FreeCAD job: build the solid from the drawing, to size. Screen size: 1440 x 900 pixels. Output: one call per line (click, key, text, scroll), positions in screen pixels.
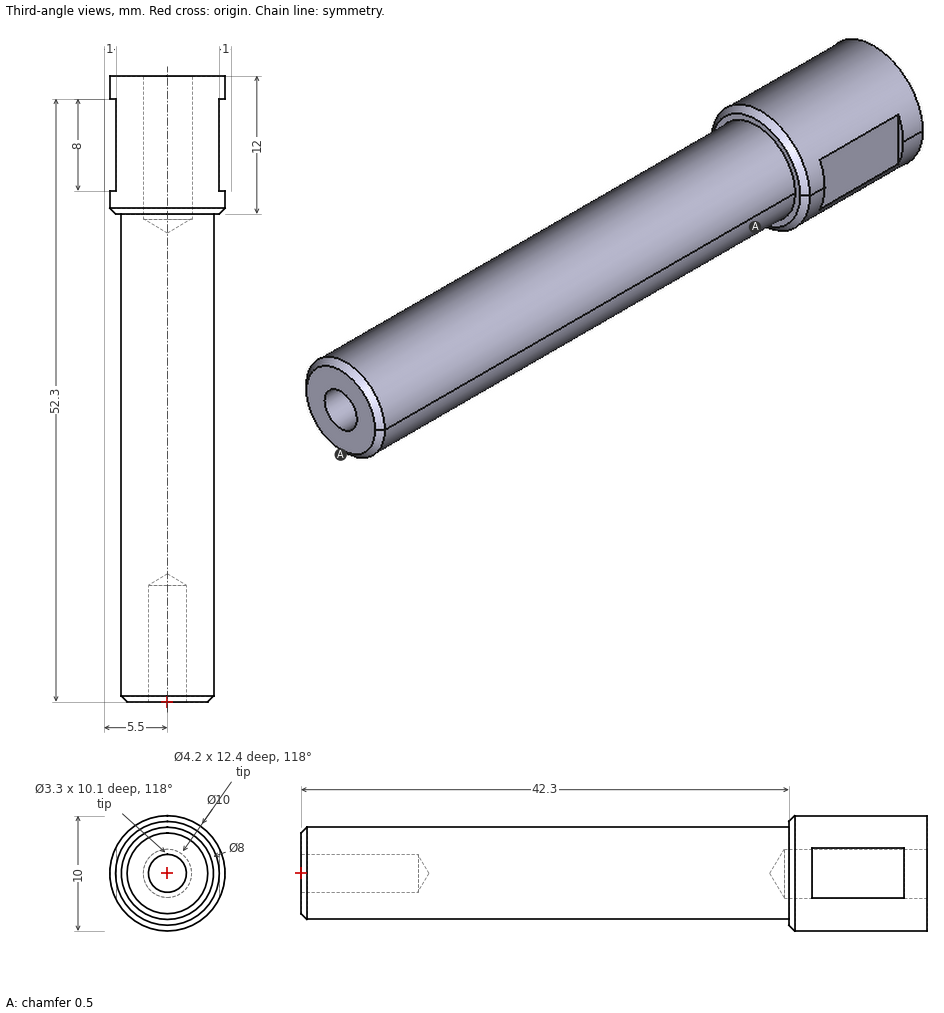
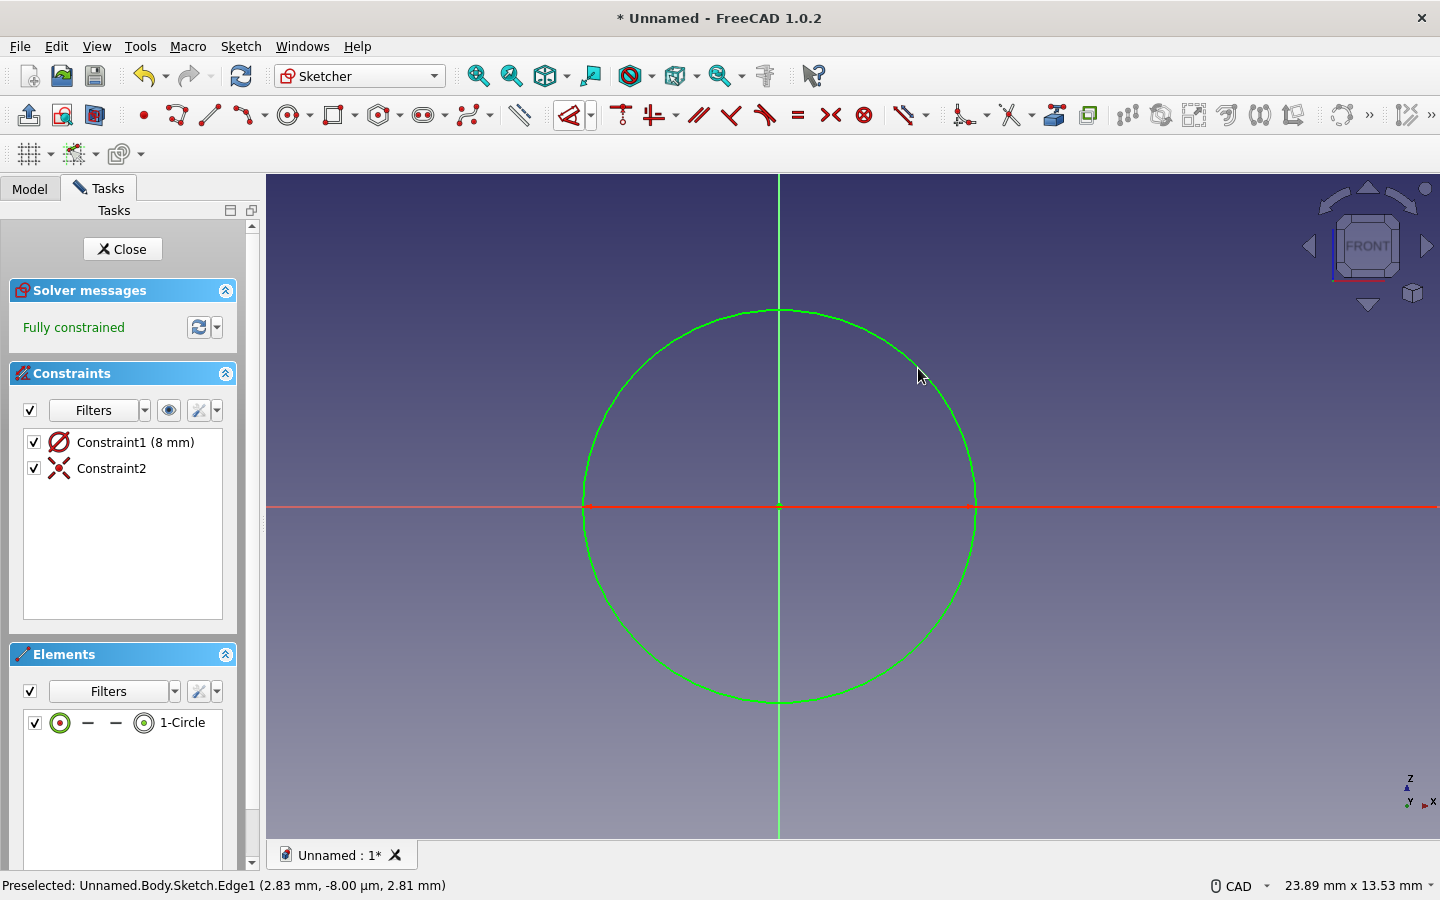
click(123, 249)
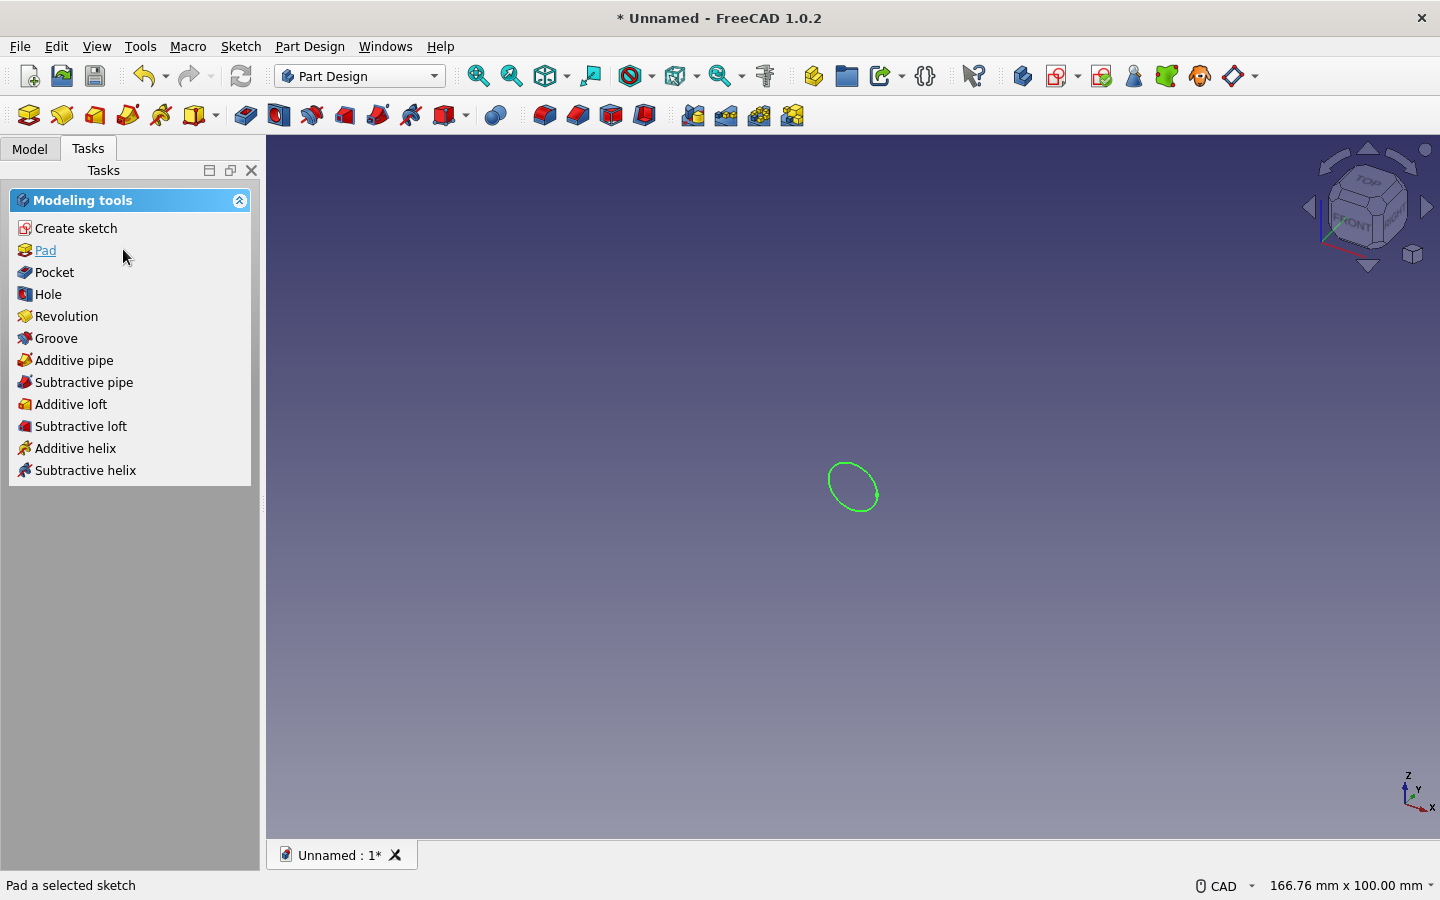
click(29, 116)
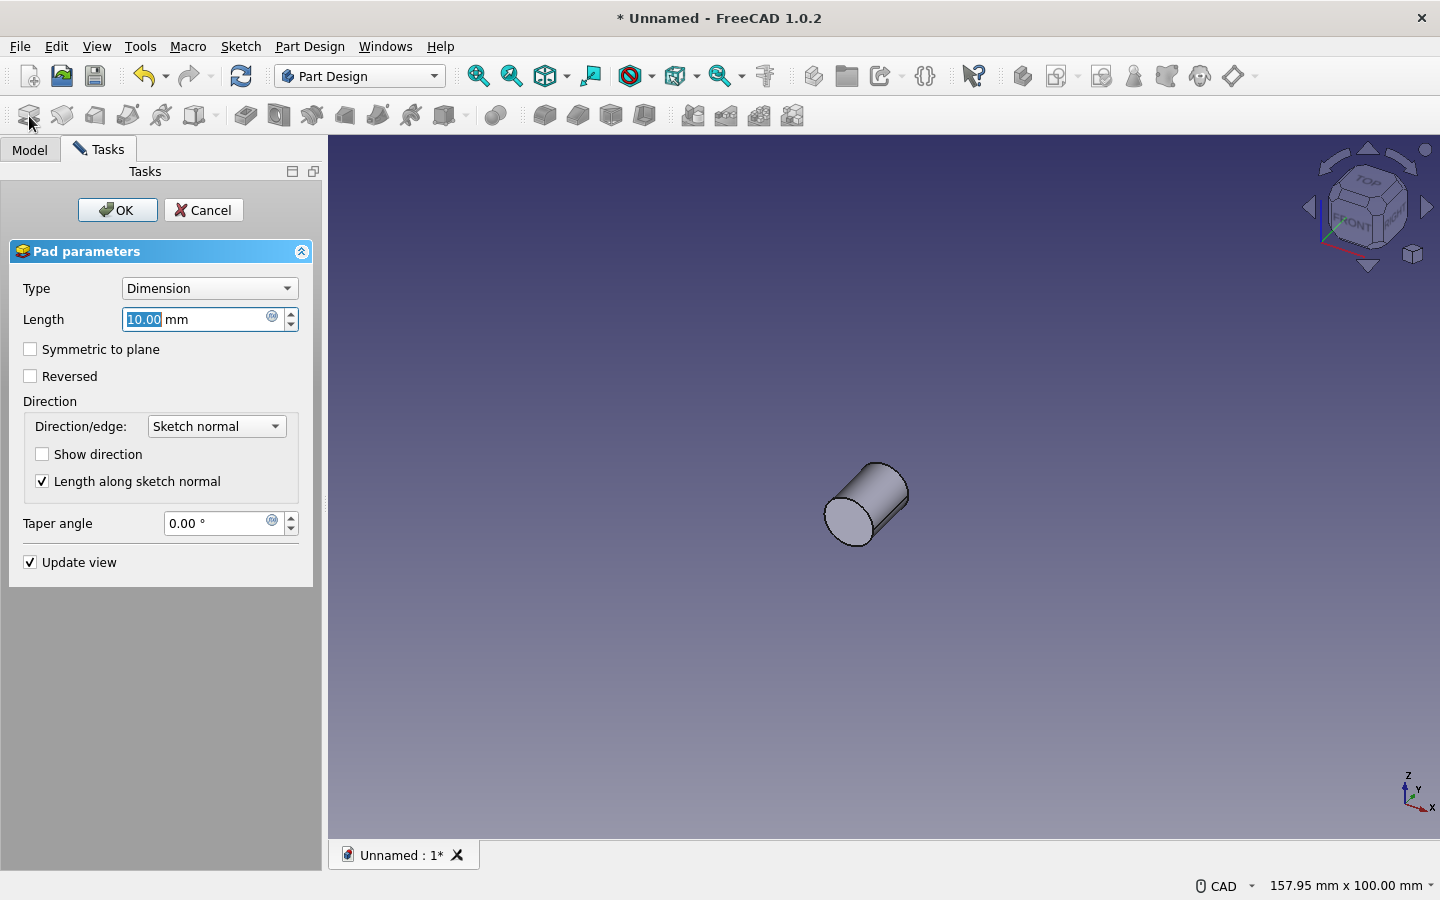
text(42.3)
key(Tab)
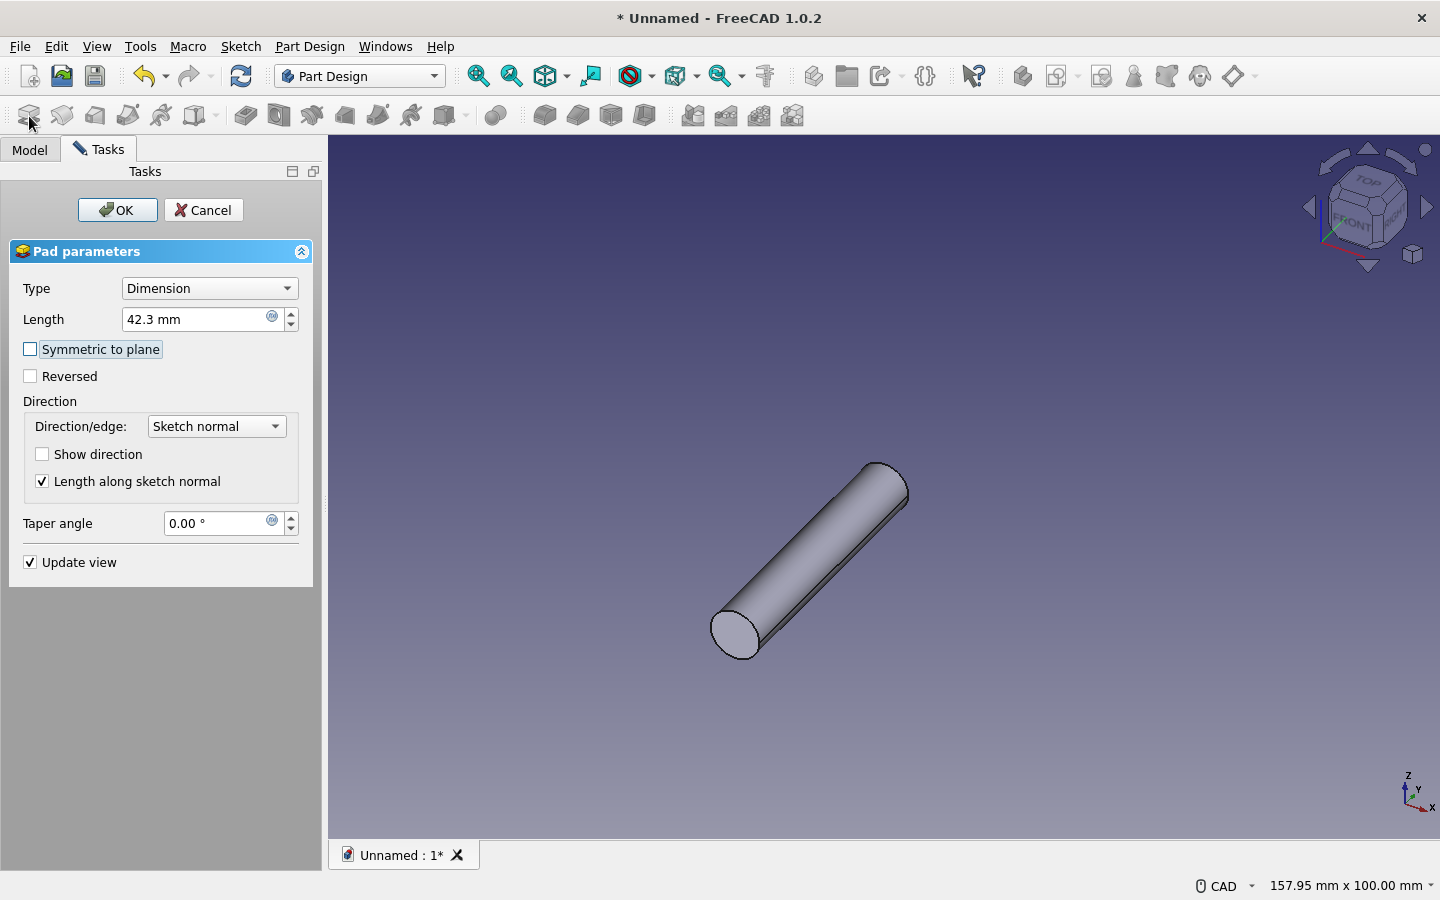
click(31, 376)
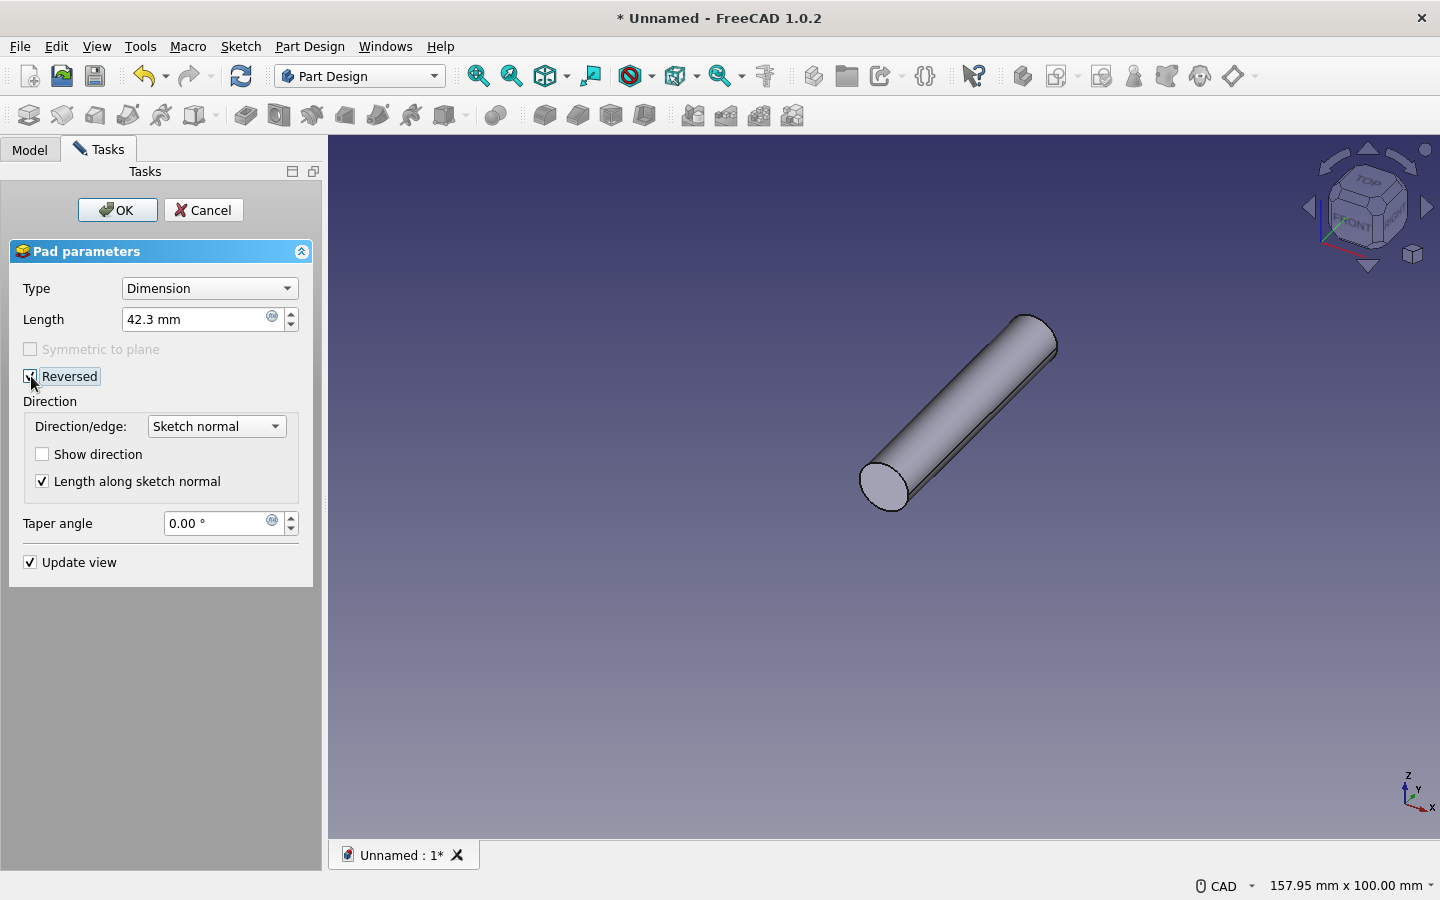
click(118, 210)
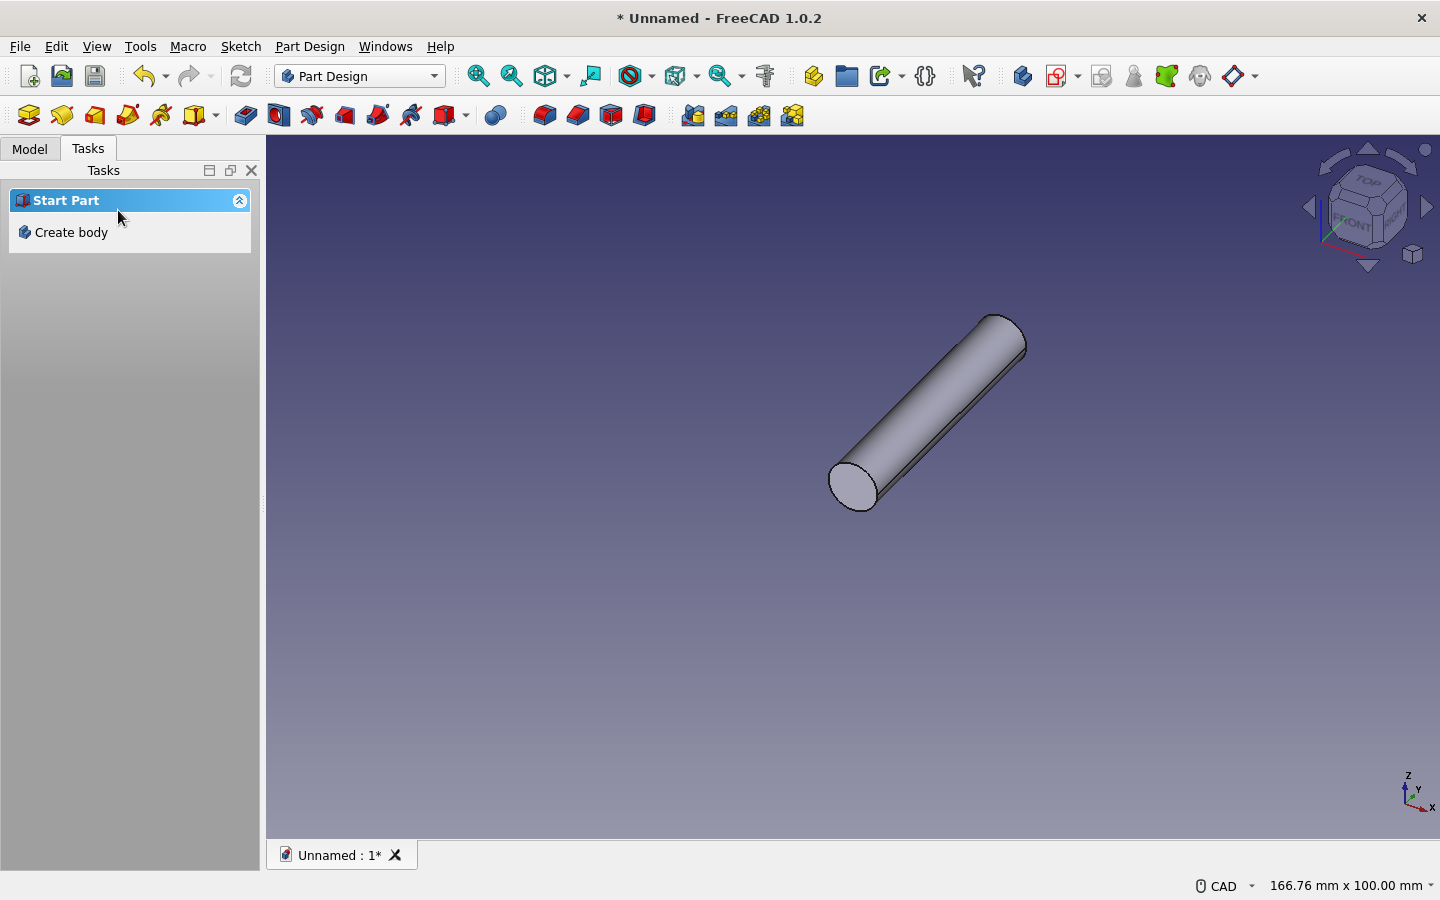
key(v)
key(f)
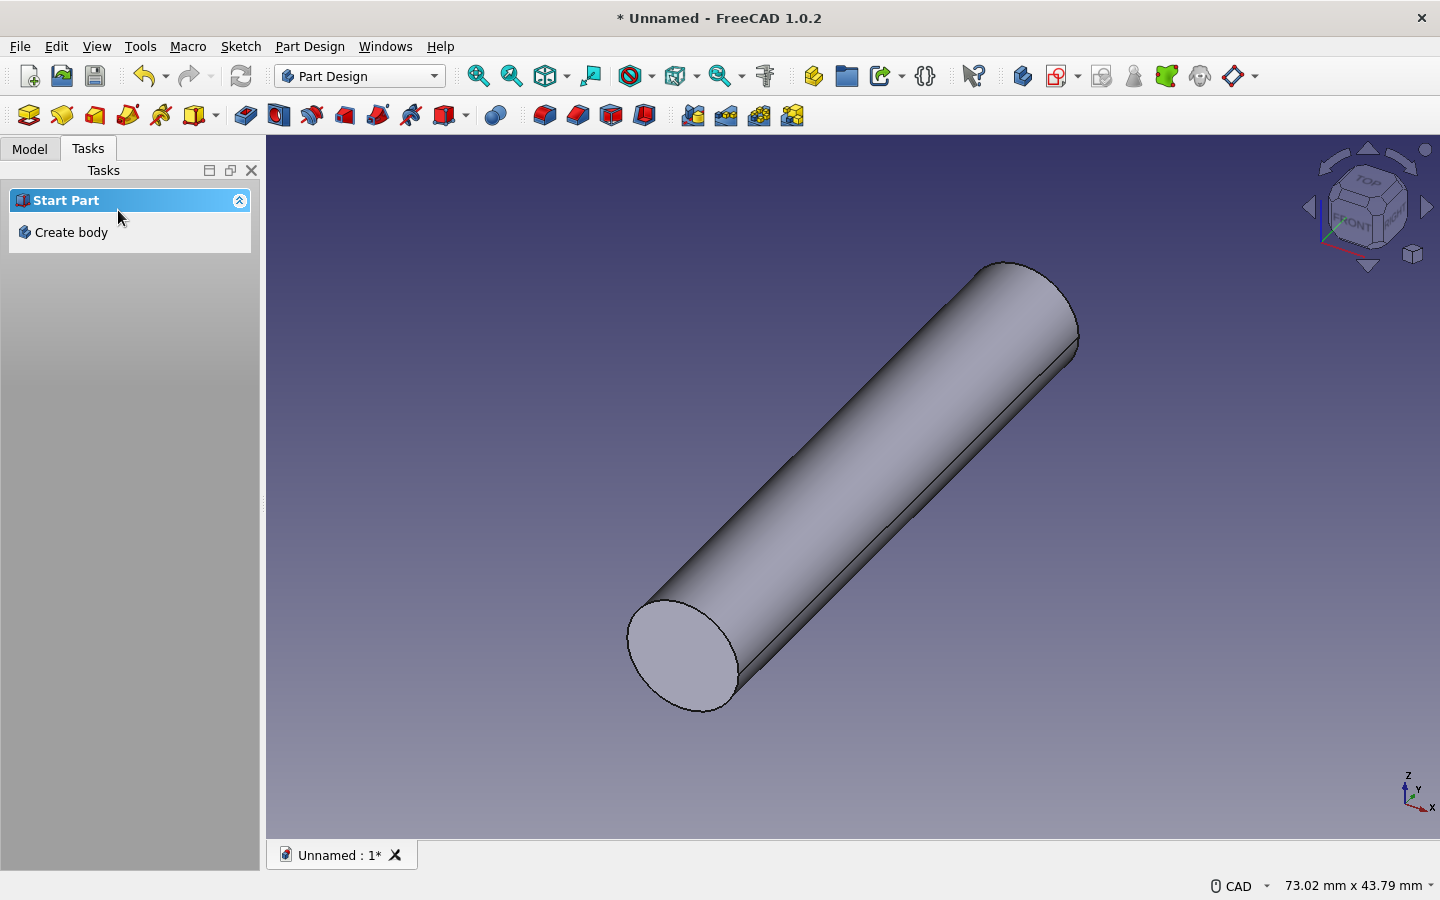
key(4)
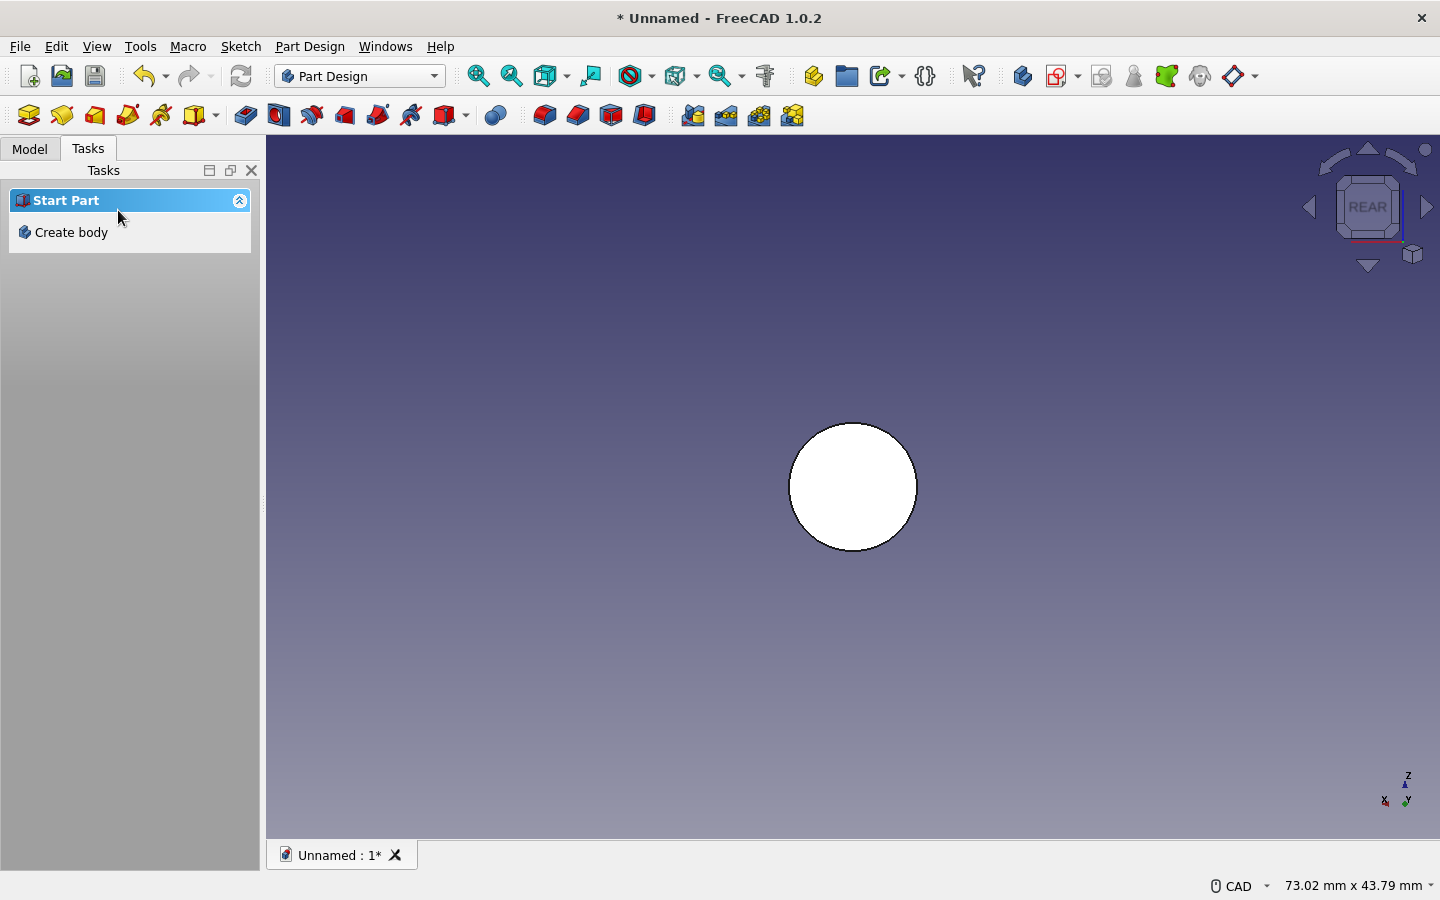
click(479, 76)